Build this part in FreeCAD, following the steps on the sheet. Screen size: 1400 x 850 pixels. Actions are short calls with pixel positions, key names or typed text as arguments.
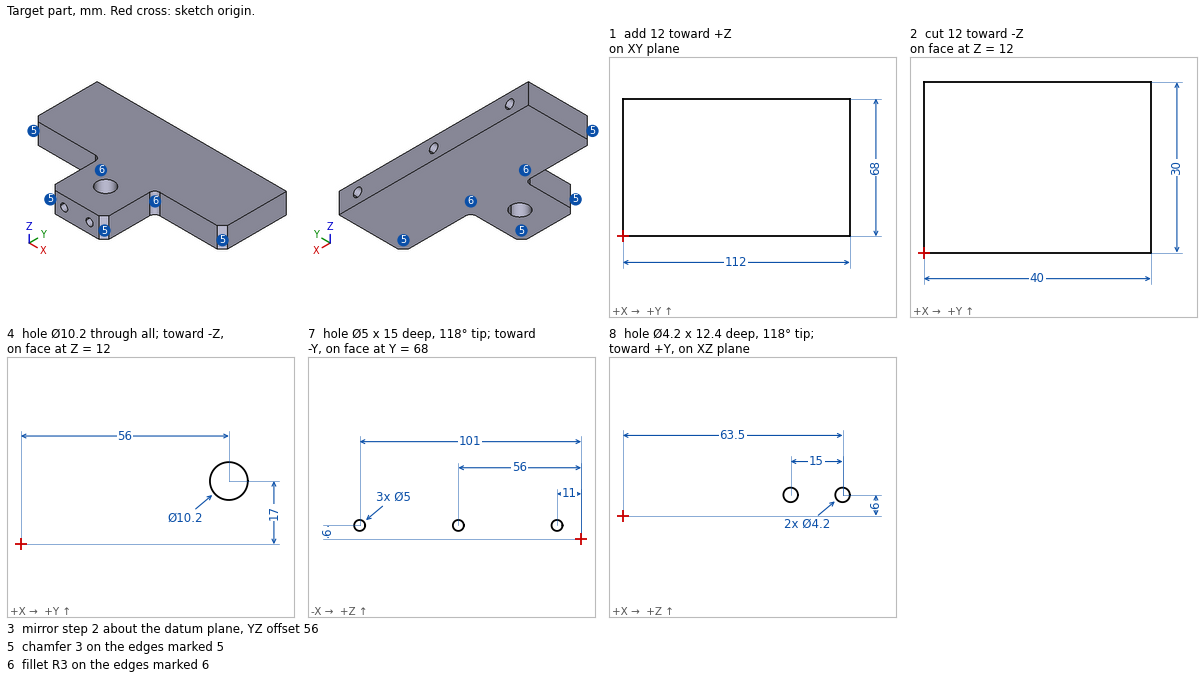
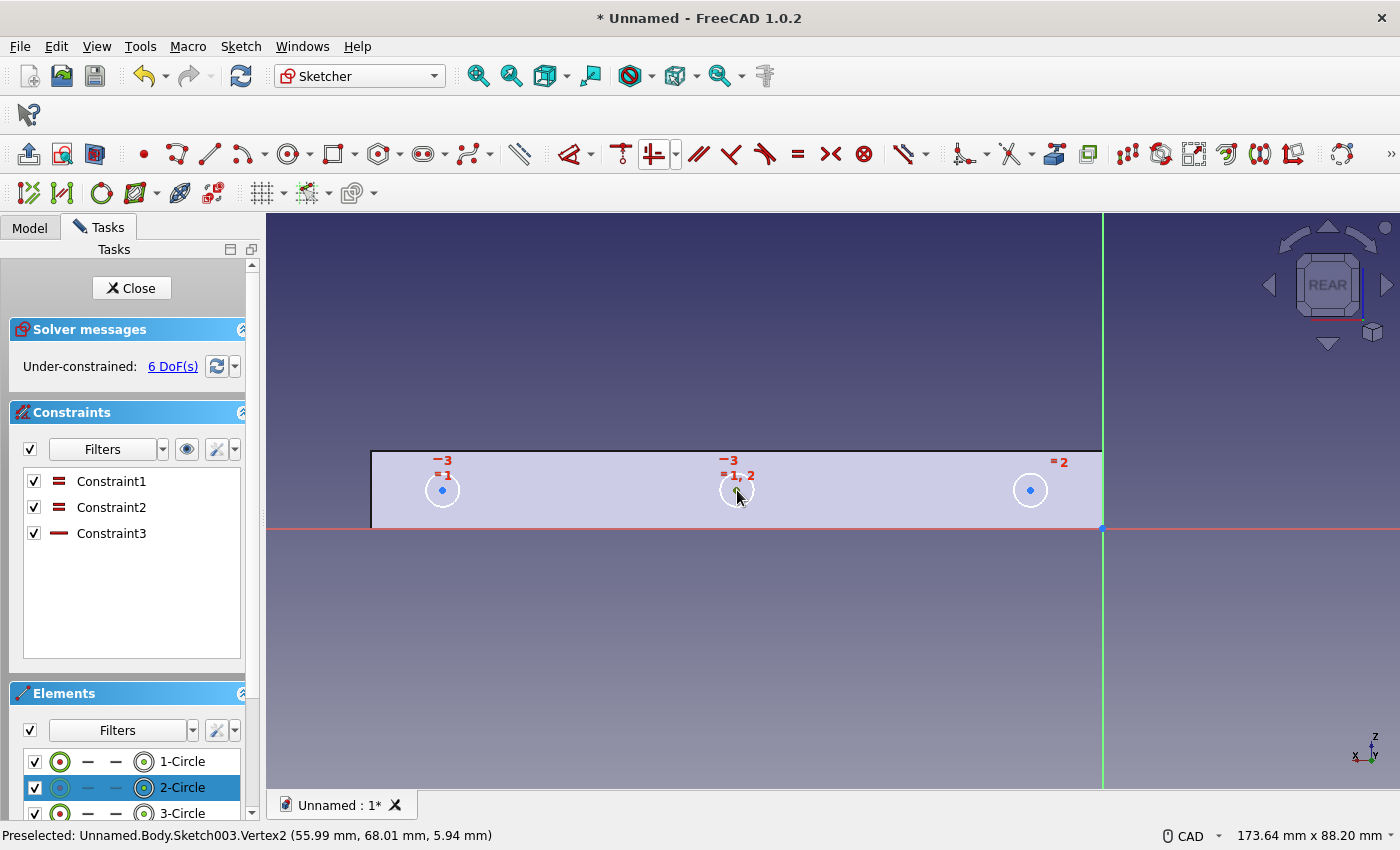
click(1031, 490)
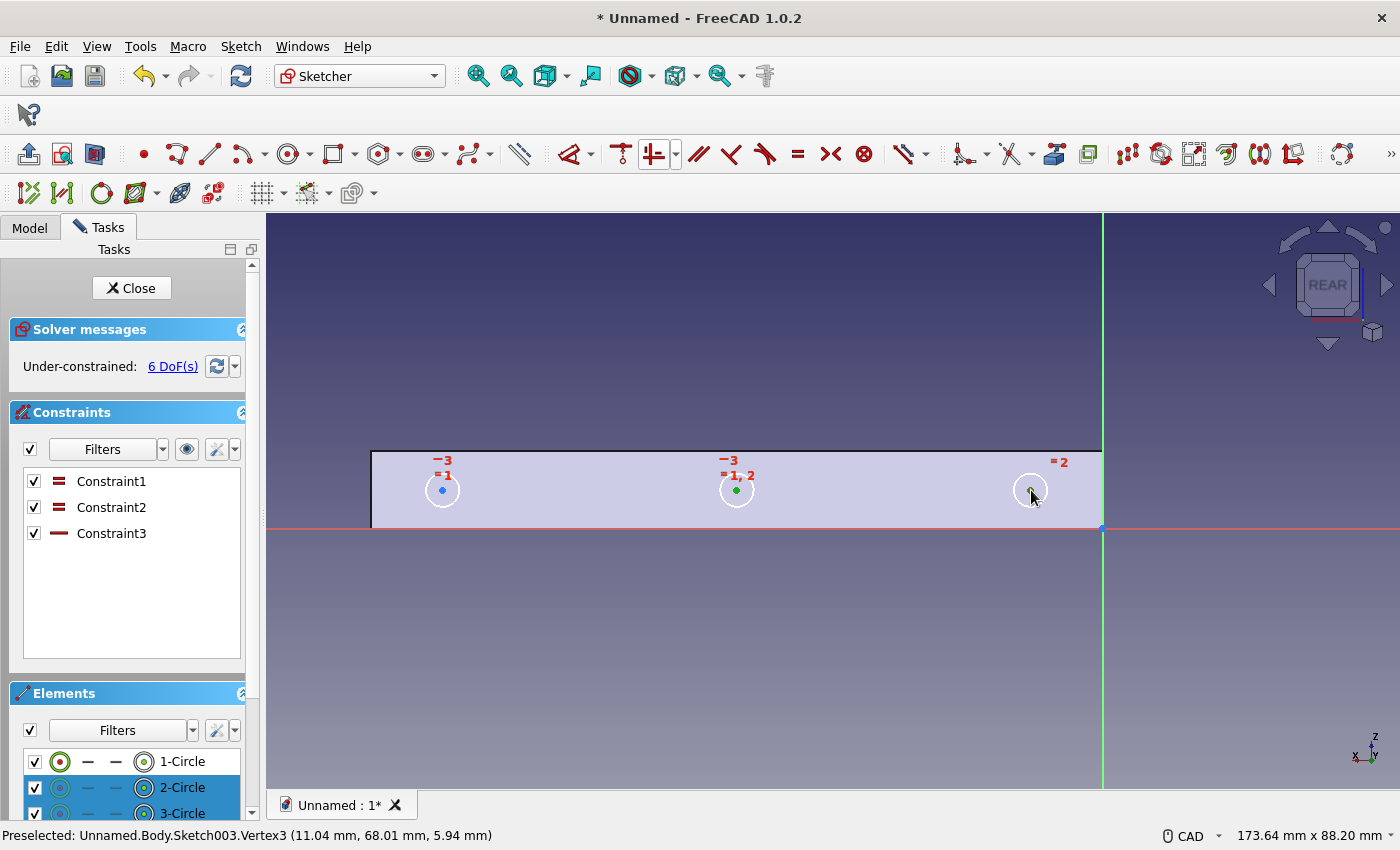
key(h)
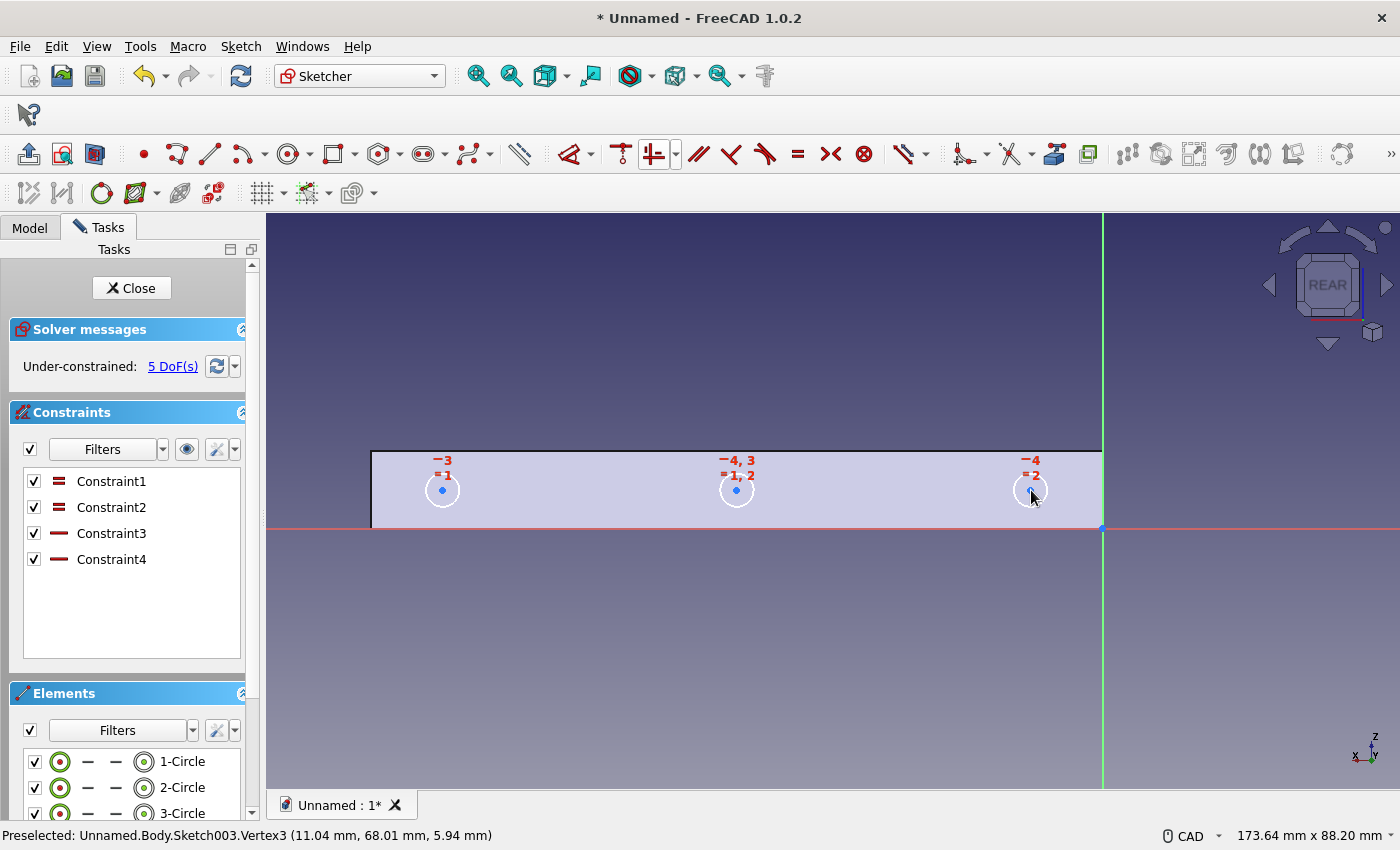
click(568, 154)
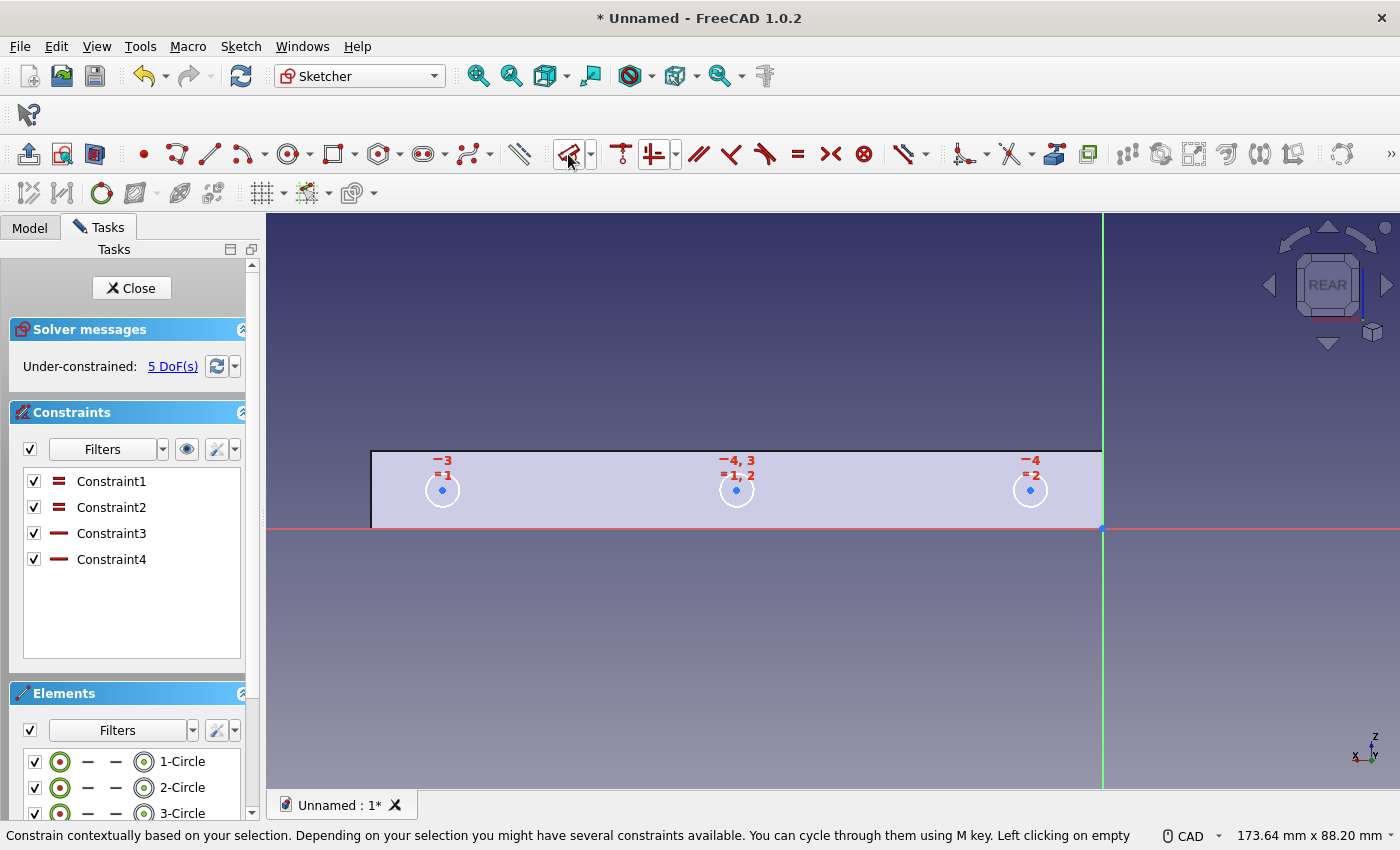
click(454, 478)
click(476, 455)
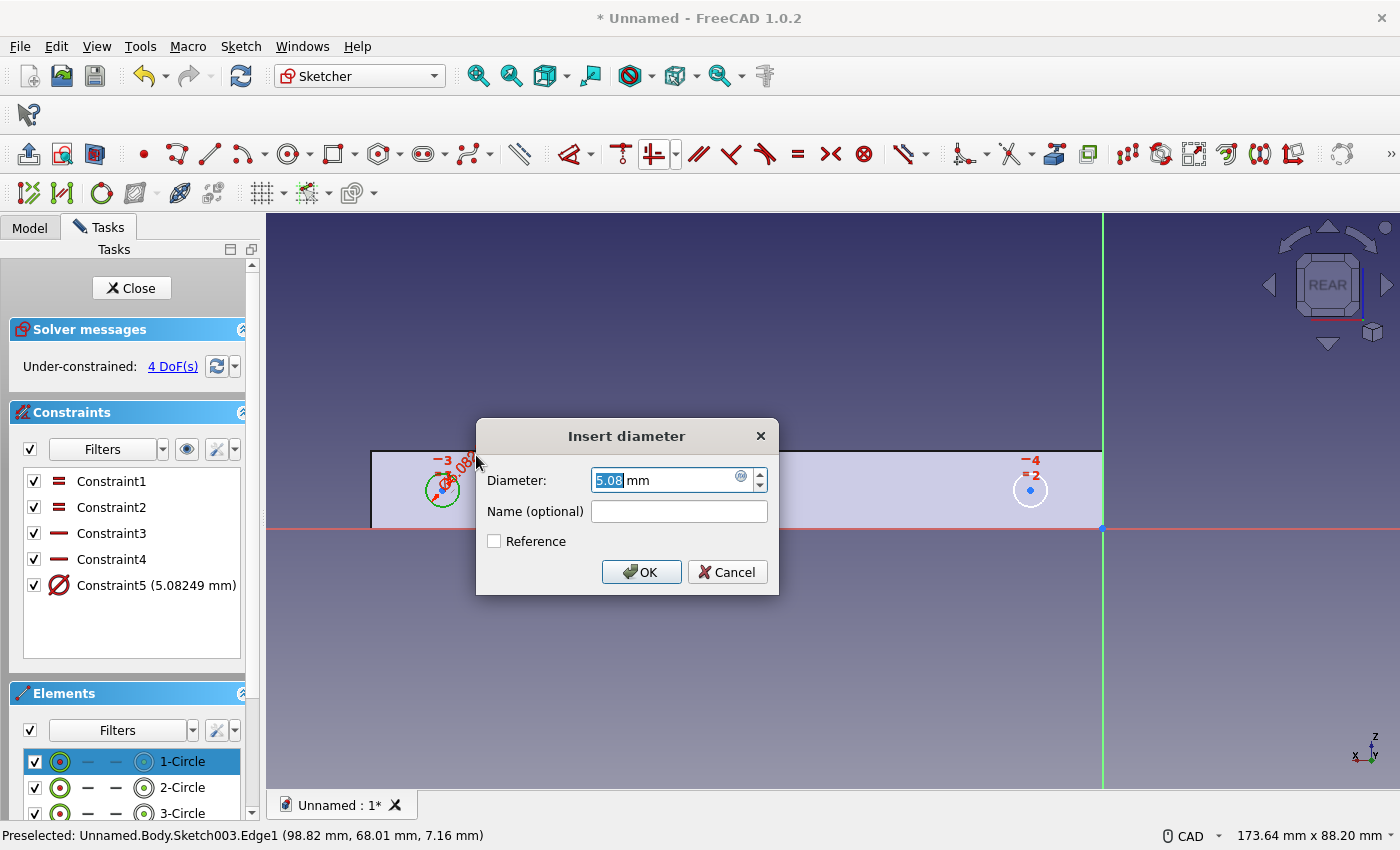
text(5)
key(Return)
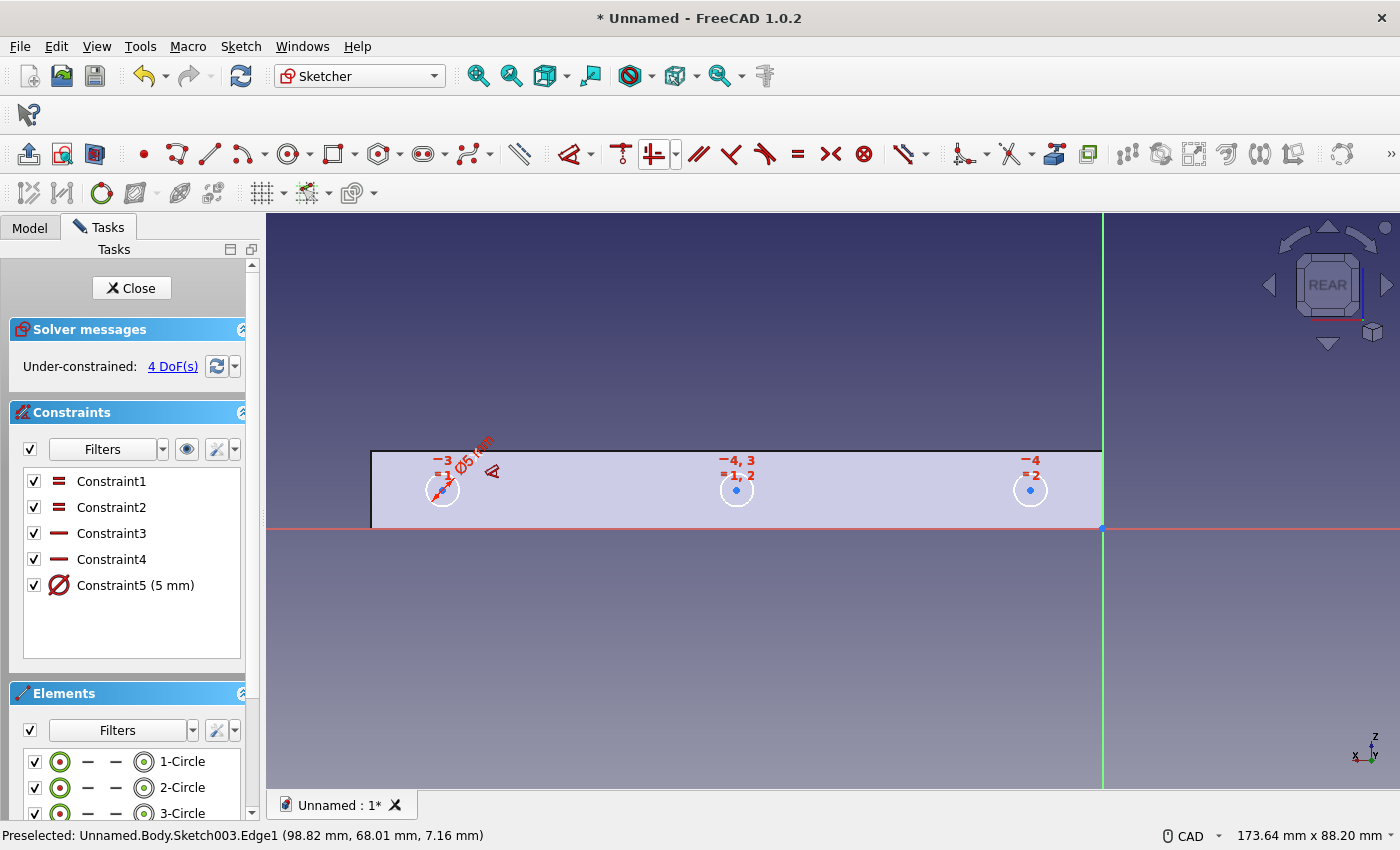
click(443, 490)
click(1137, 510)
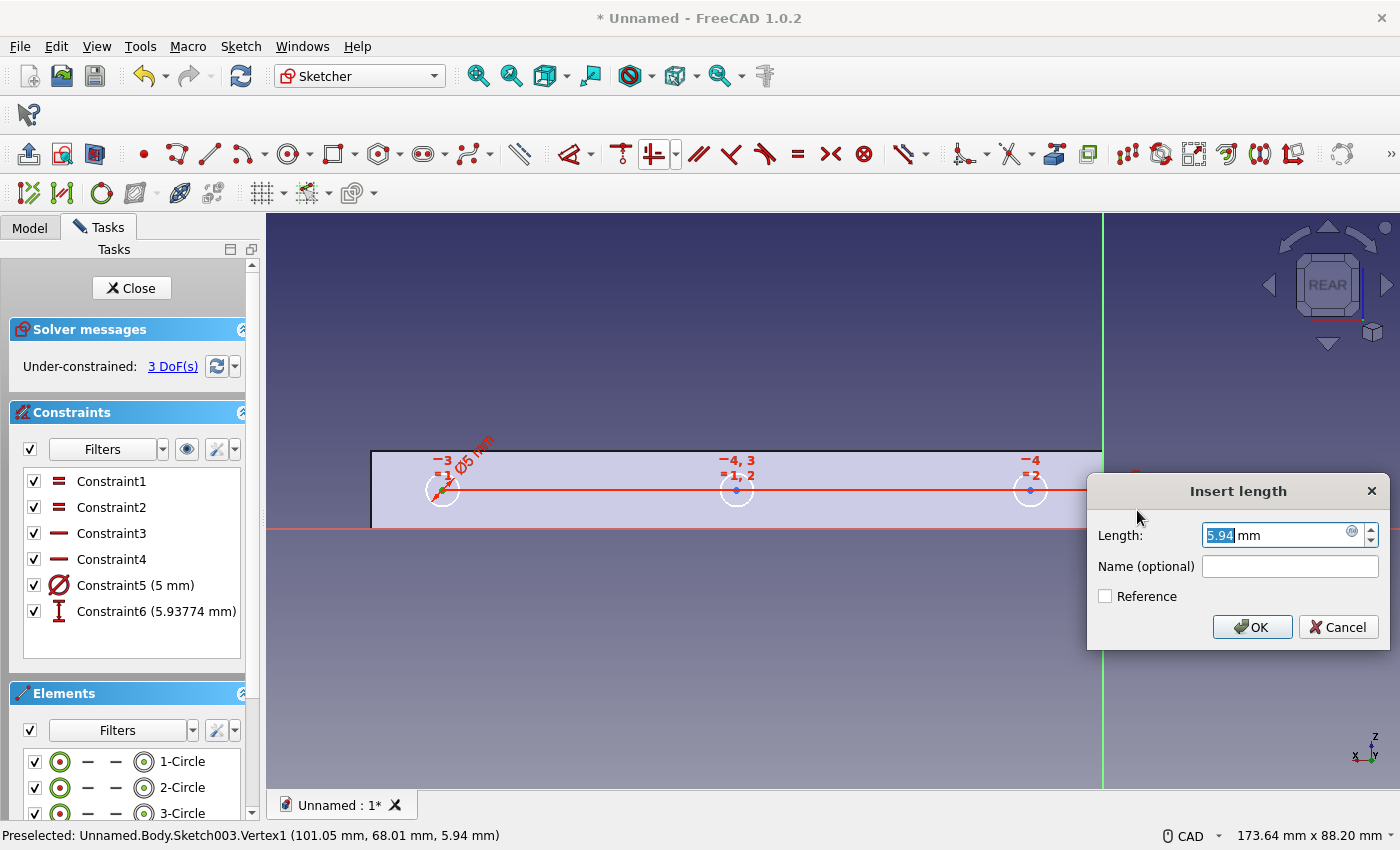
text(6)
key(Return)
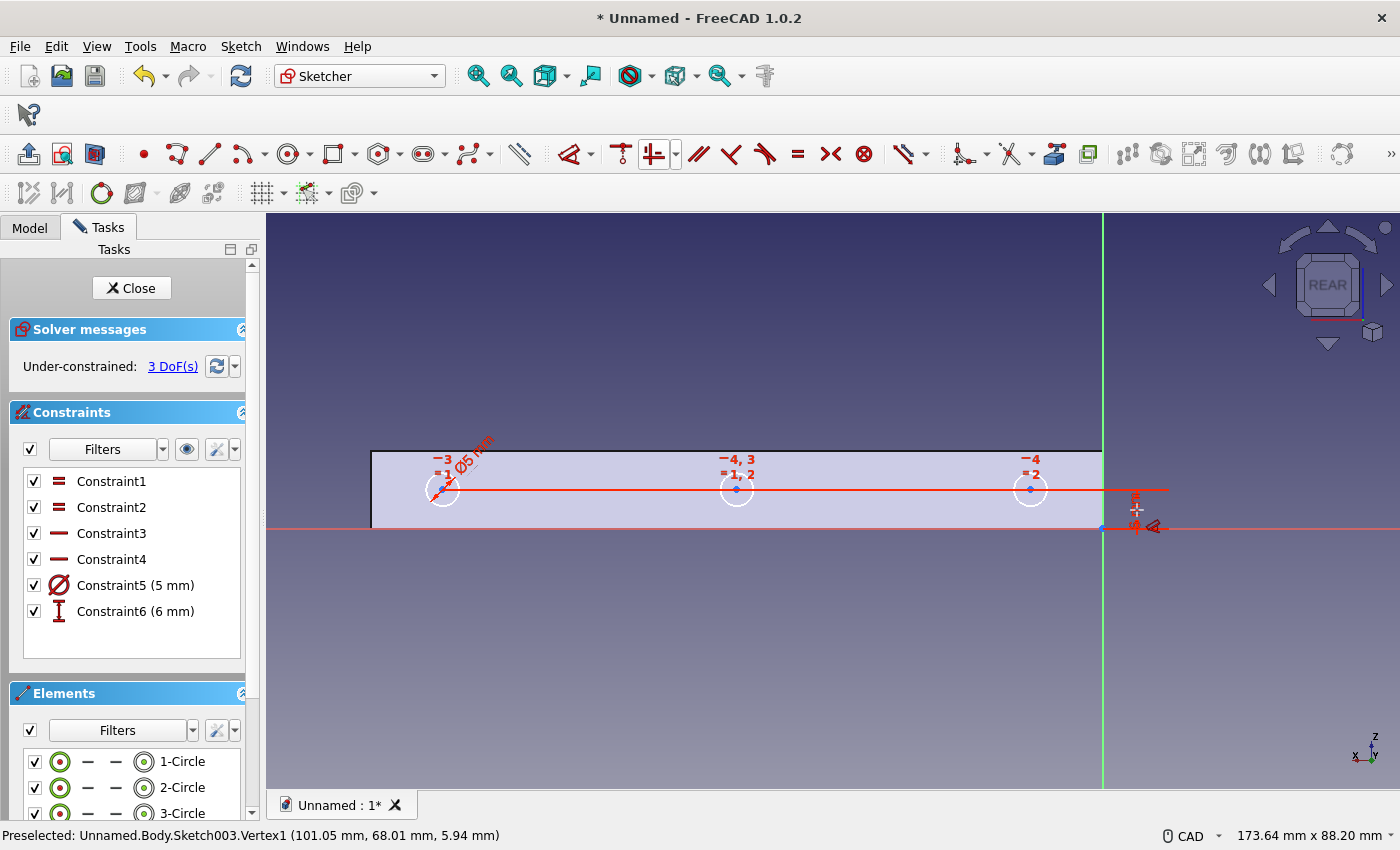
click(737, 490)
click(920, 563)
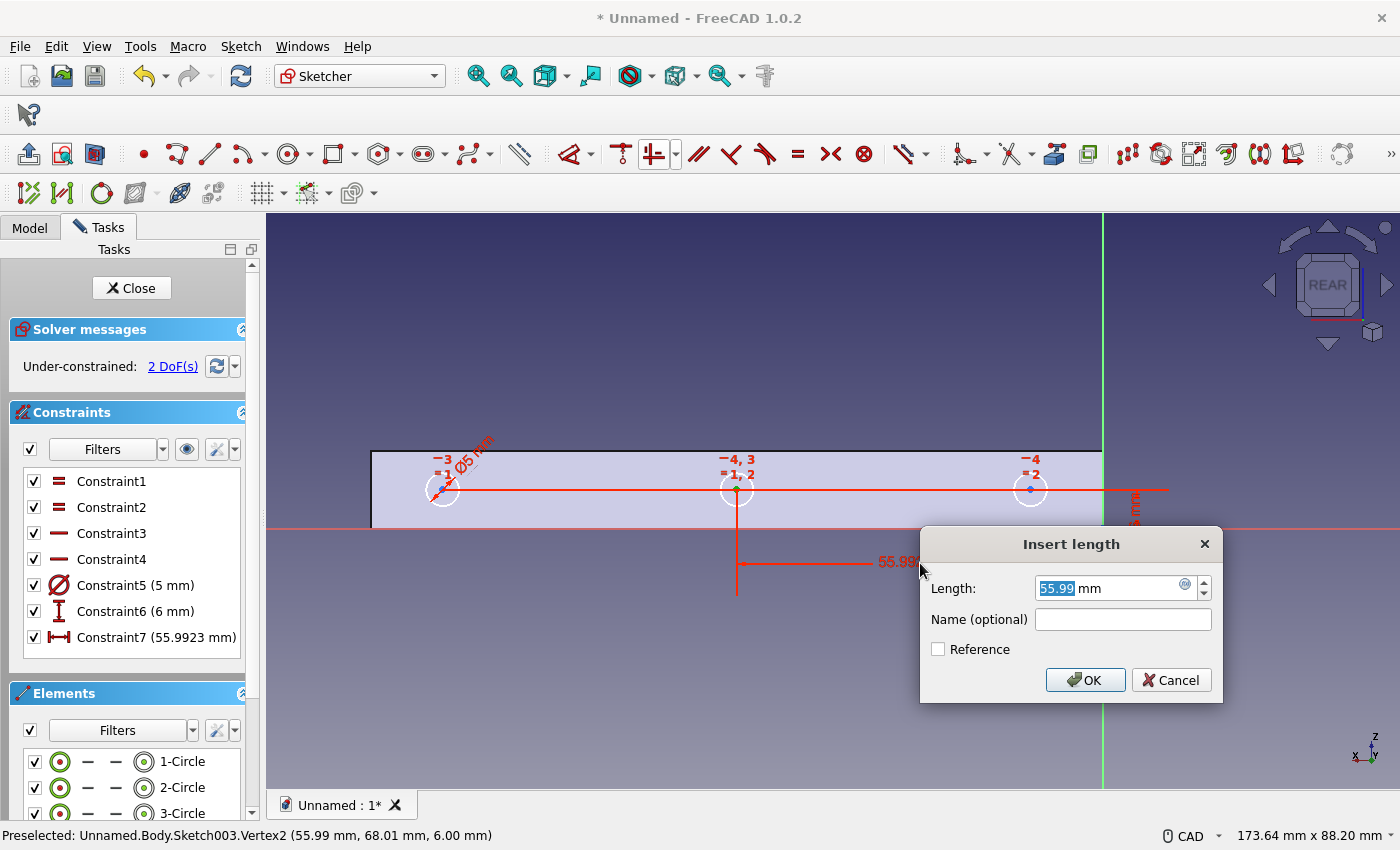
text(56)
key(Return)